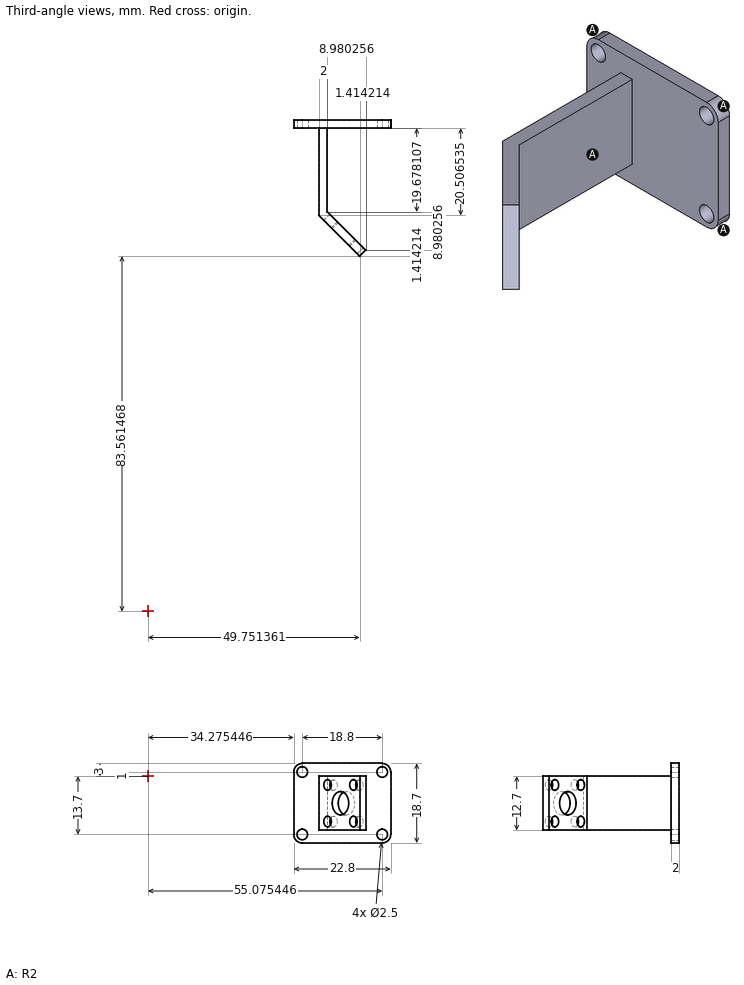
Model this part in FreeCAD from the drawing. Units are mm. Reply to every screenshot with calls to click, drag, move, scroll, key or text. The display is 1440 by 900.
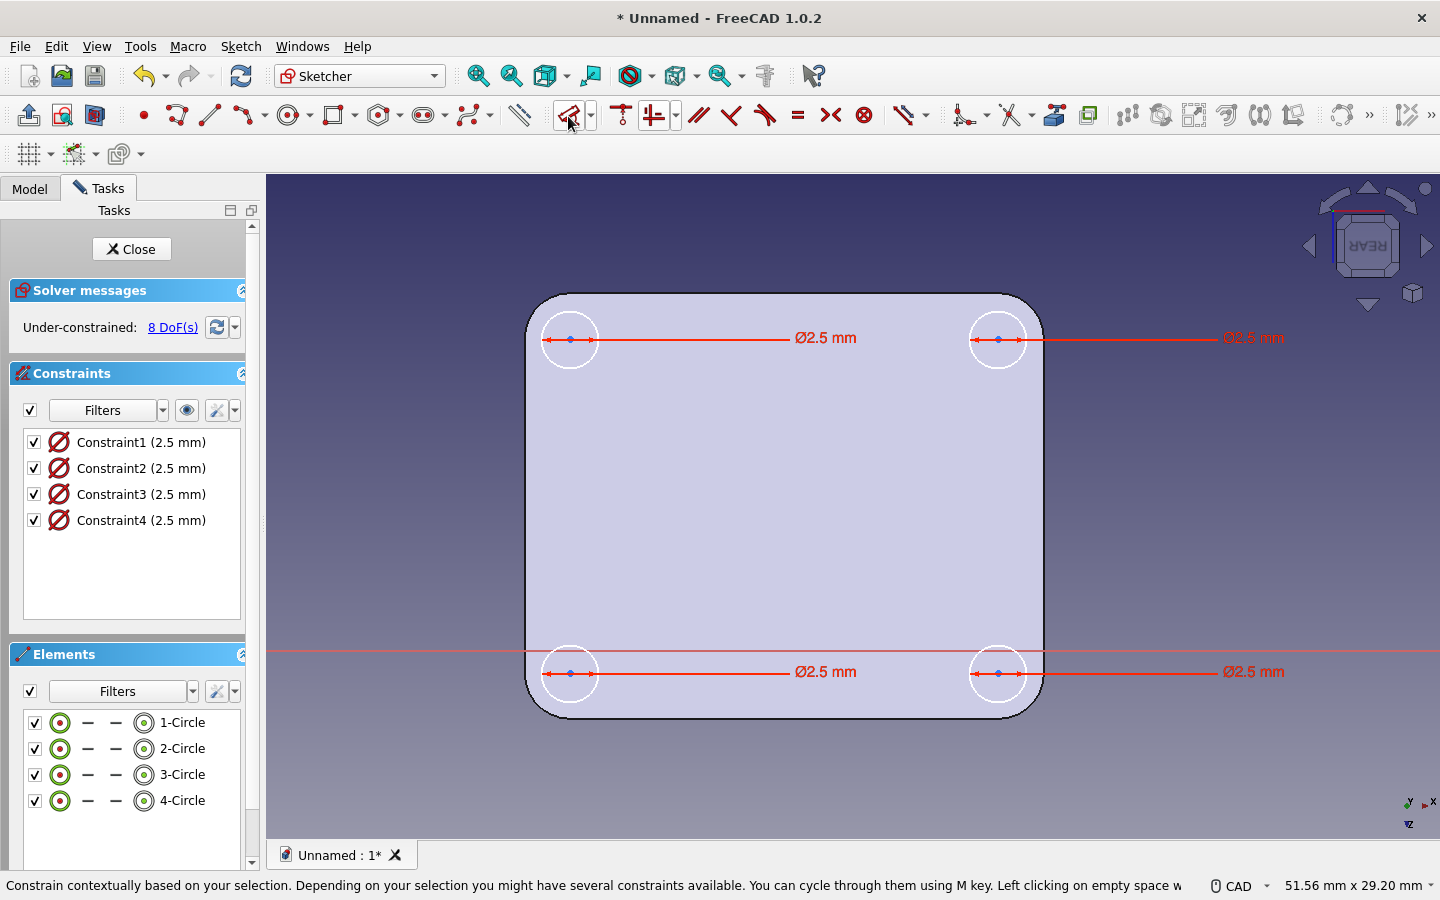
scroll(998, 674, up, 3)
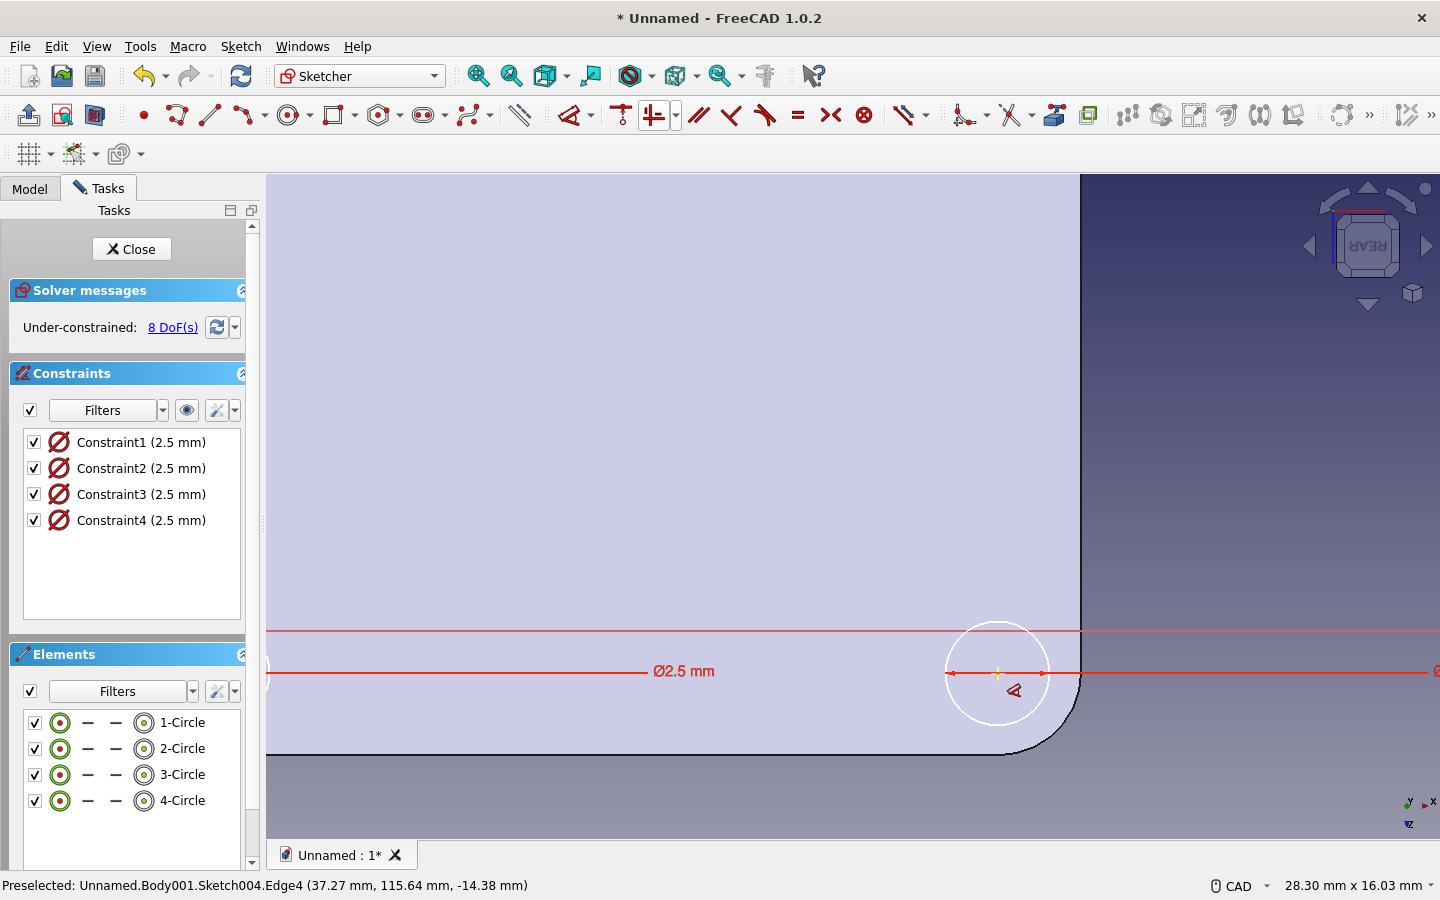
click(997, 673)
click(1031, 662)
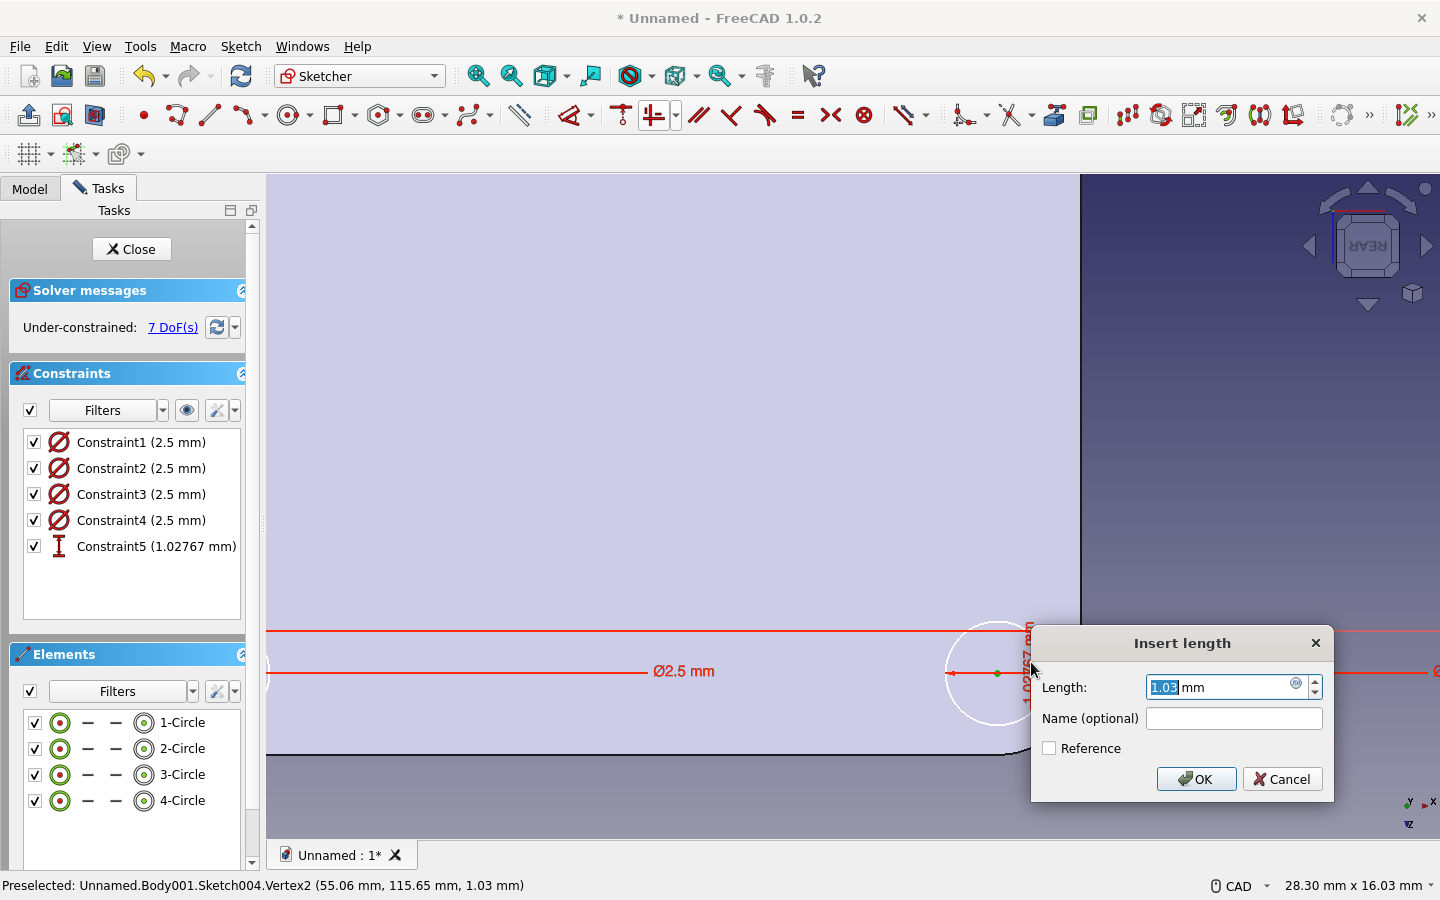
text(1)
key(Return)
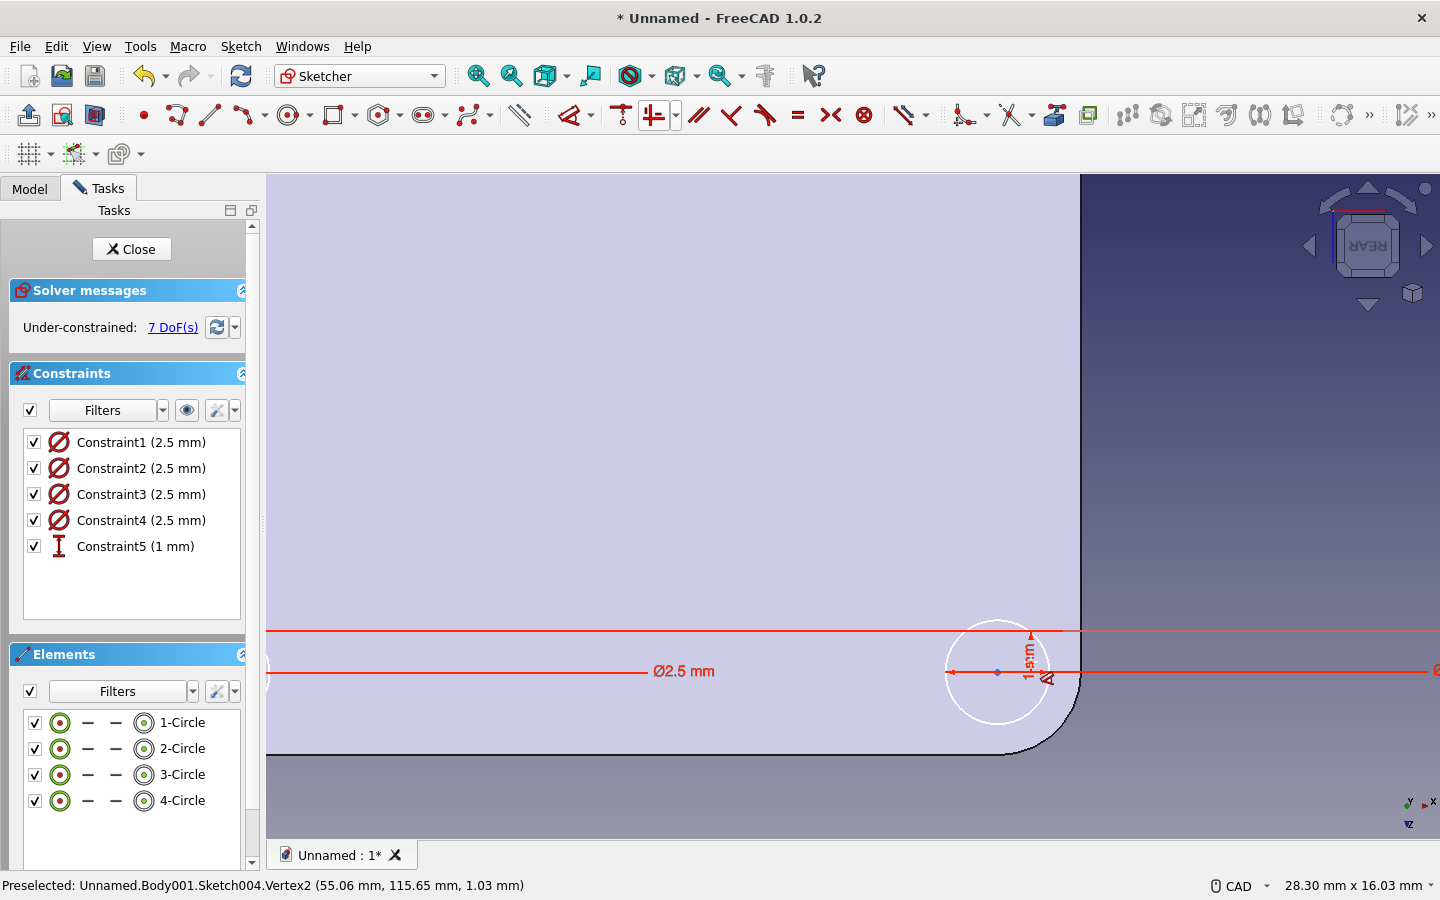
scroll(999, 676, down, 3)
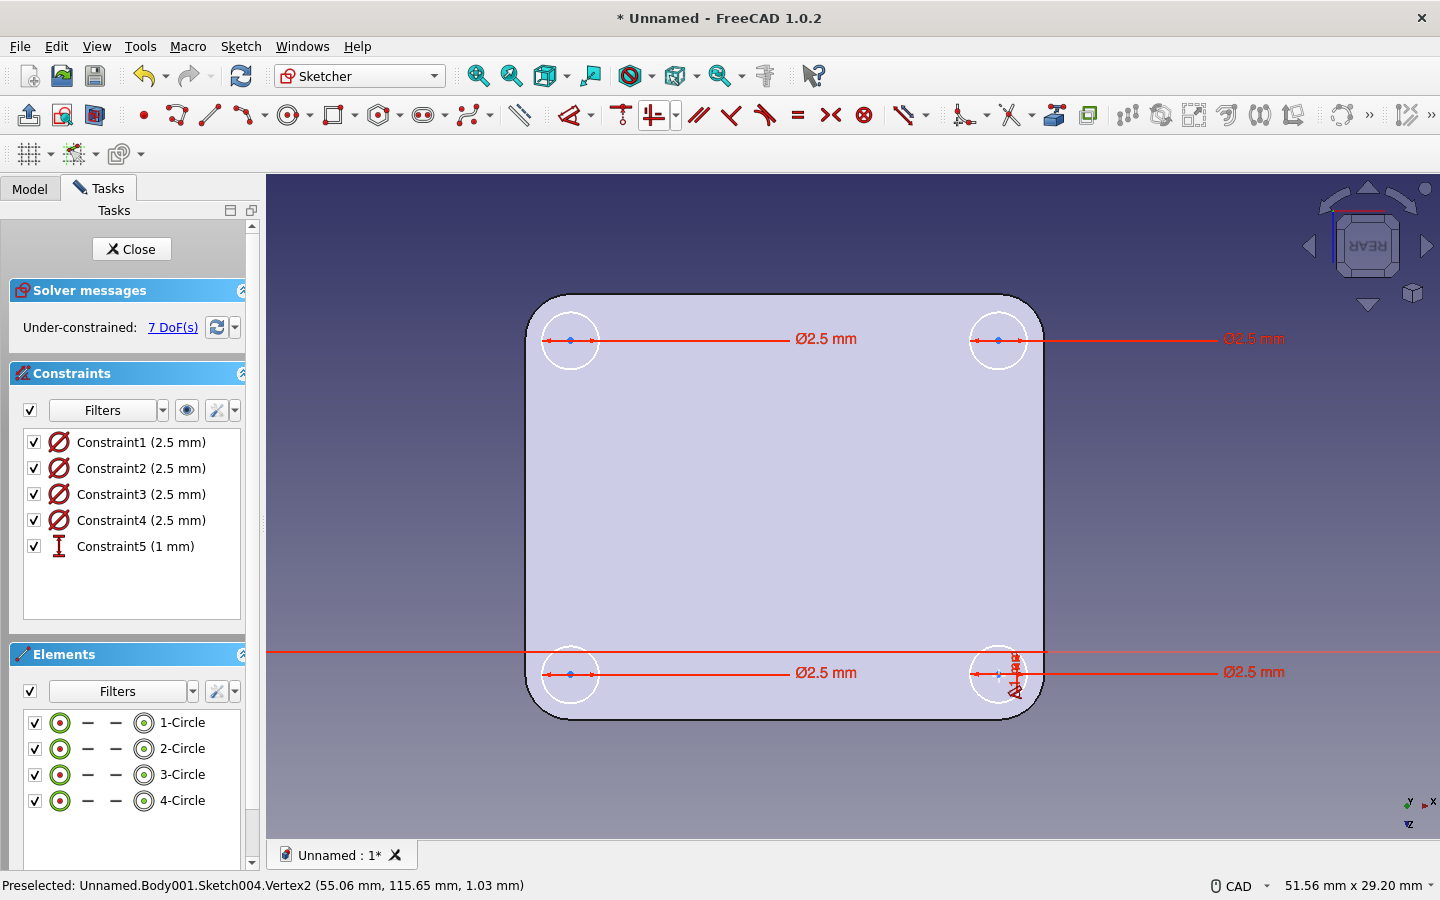
scroll(570, 675, up, 3)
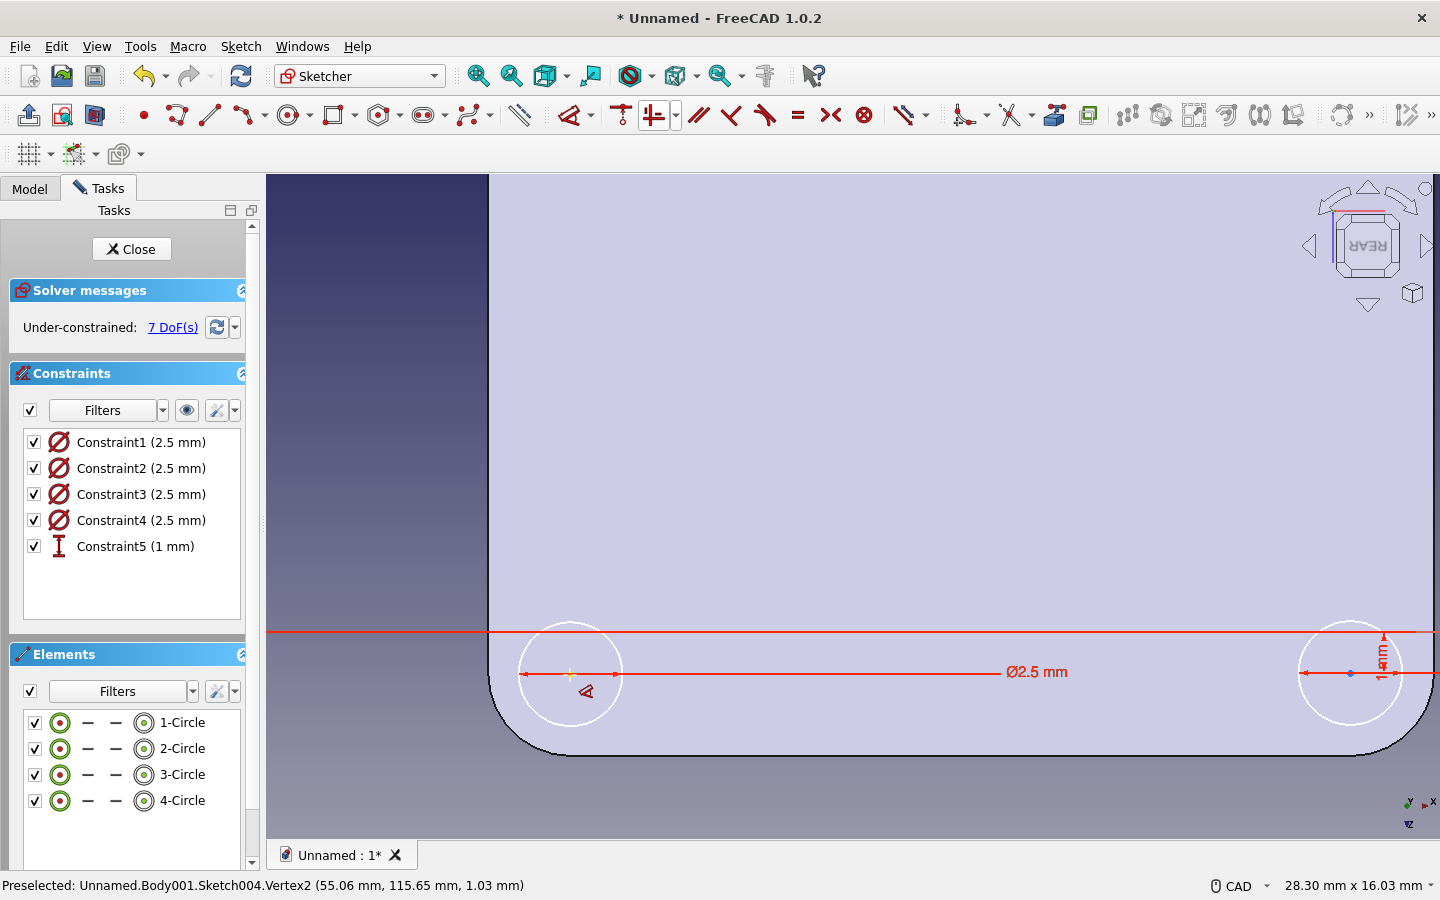
click(571, 674)
click(605, 663)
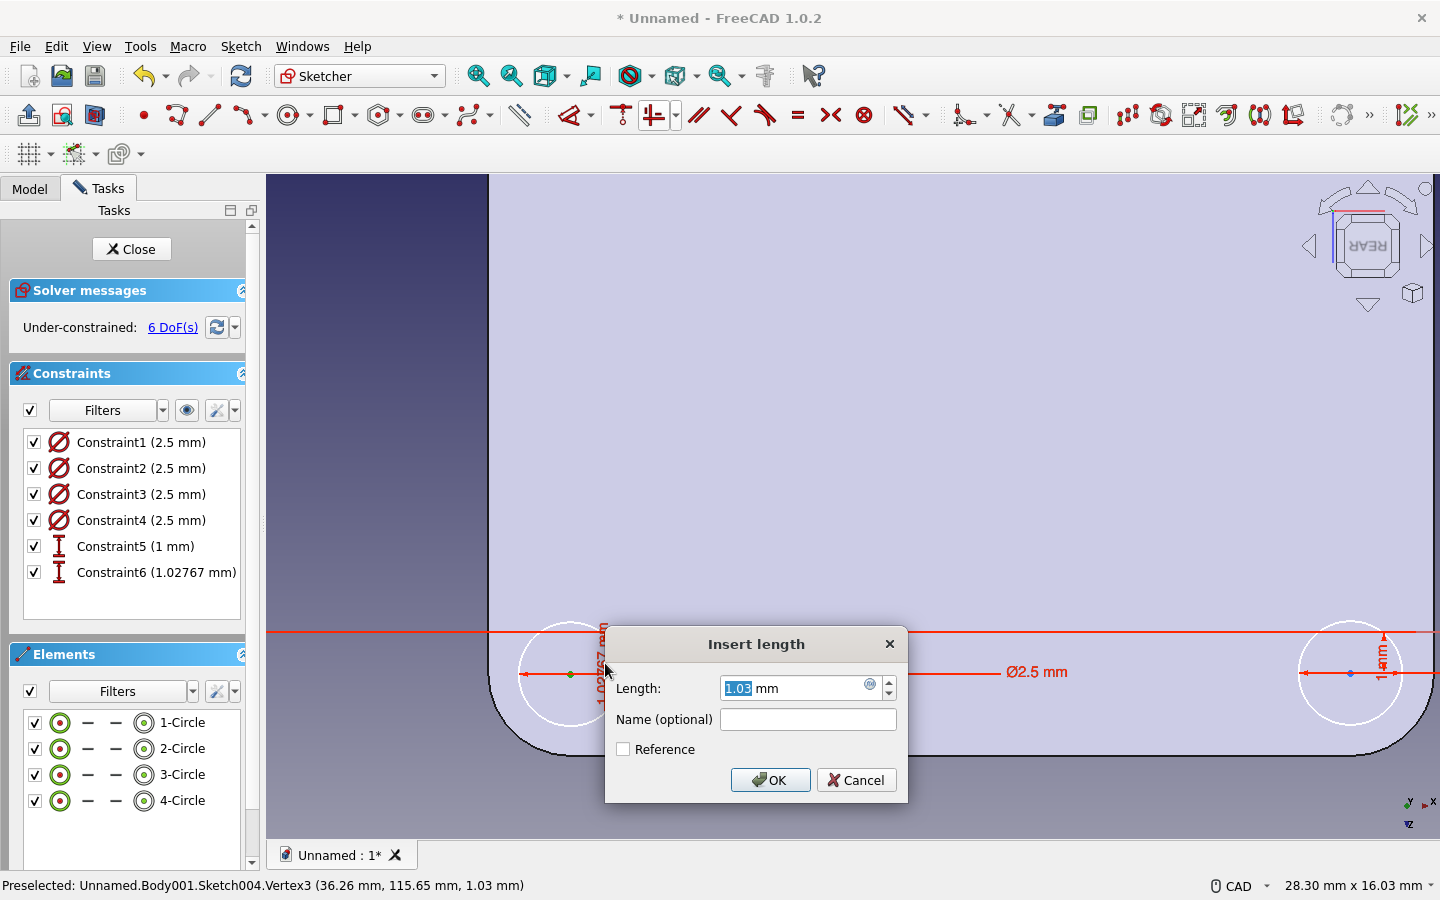
text(1)
key(Return)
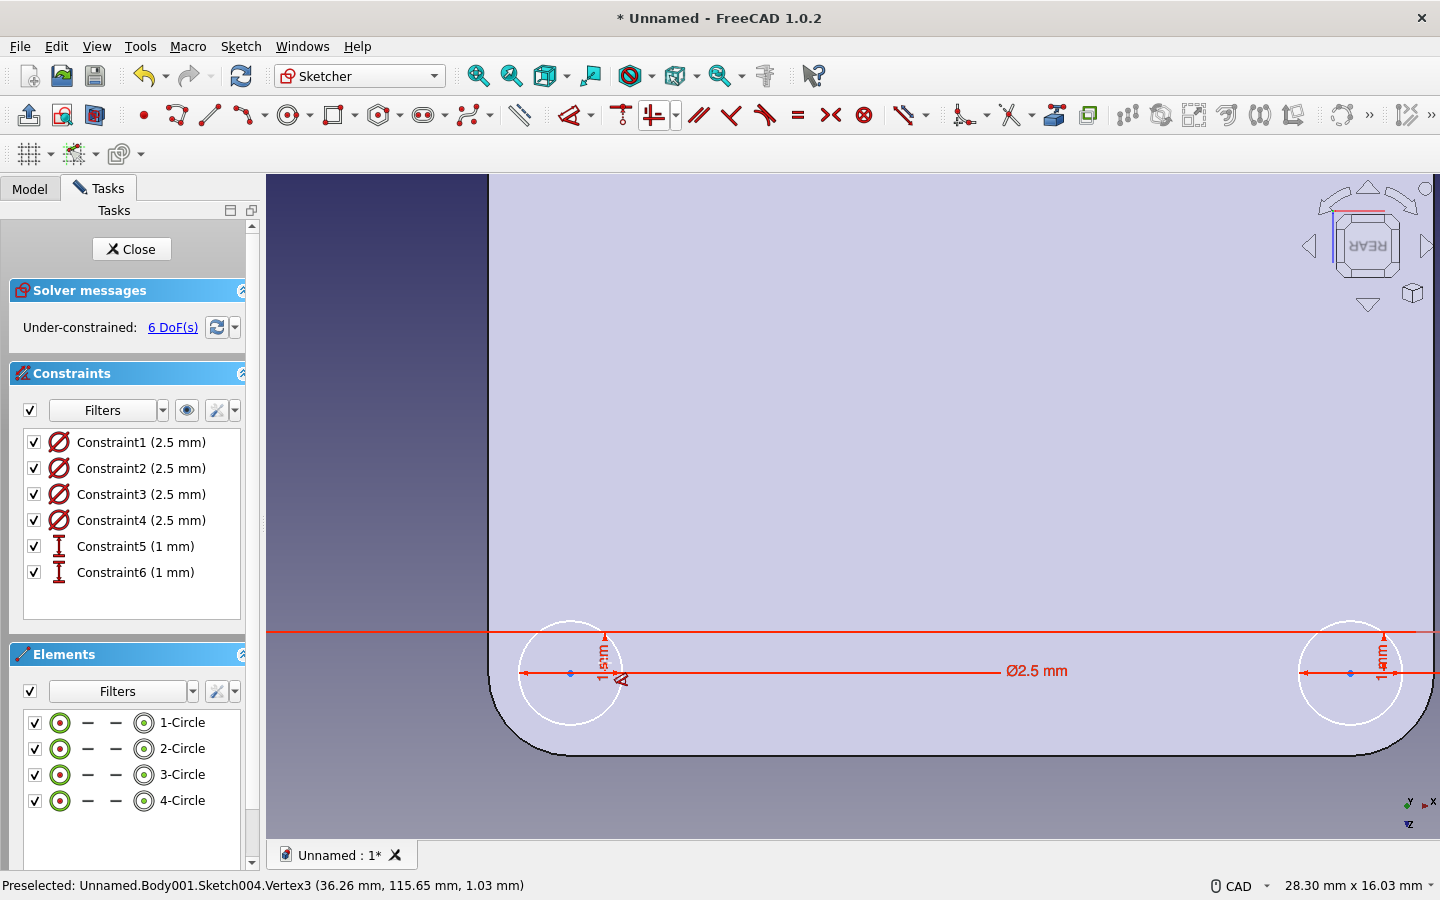
scroll(570, 675, down, 3)